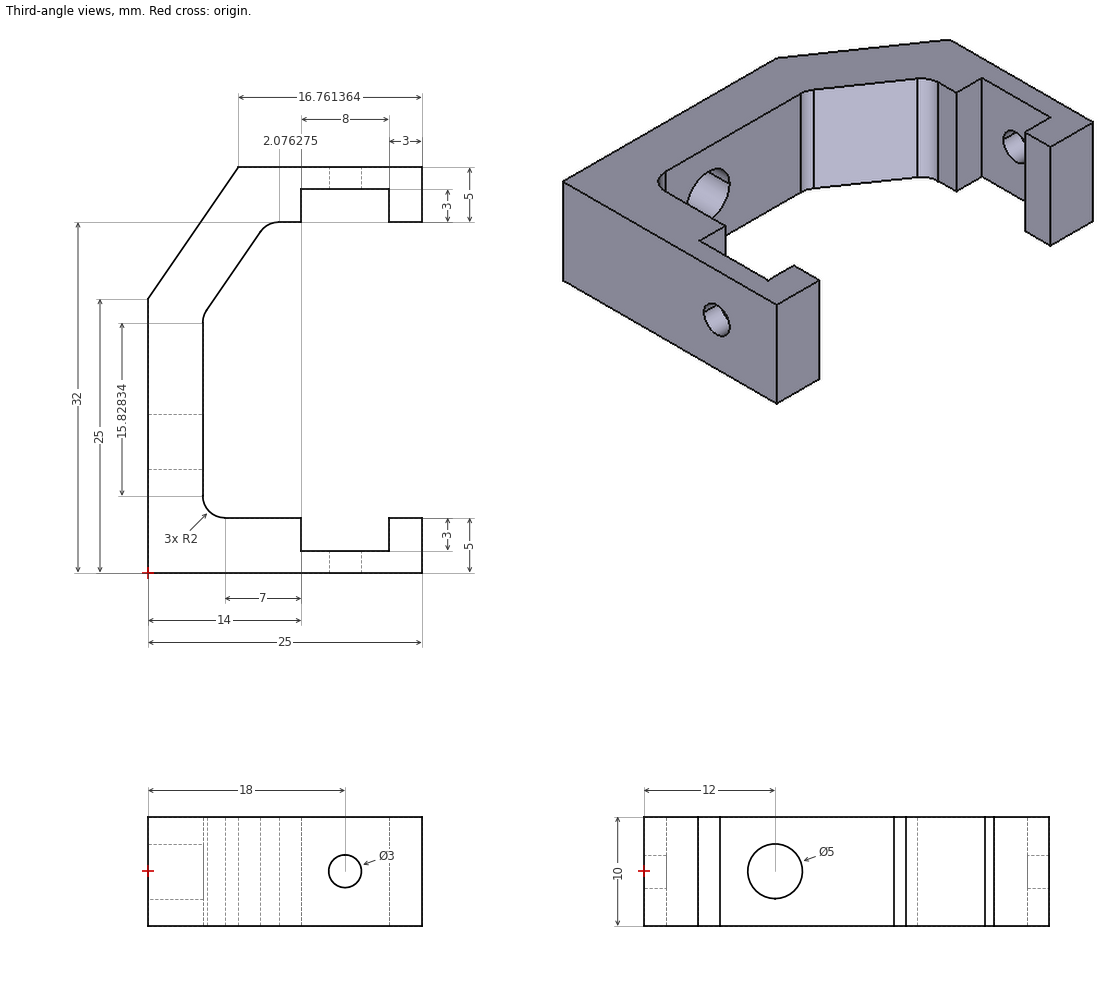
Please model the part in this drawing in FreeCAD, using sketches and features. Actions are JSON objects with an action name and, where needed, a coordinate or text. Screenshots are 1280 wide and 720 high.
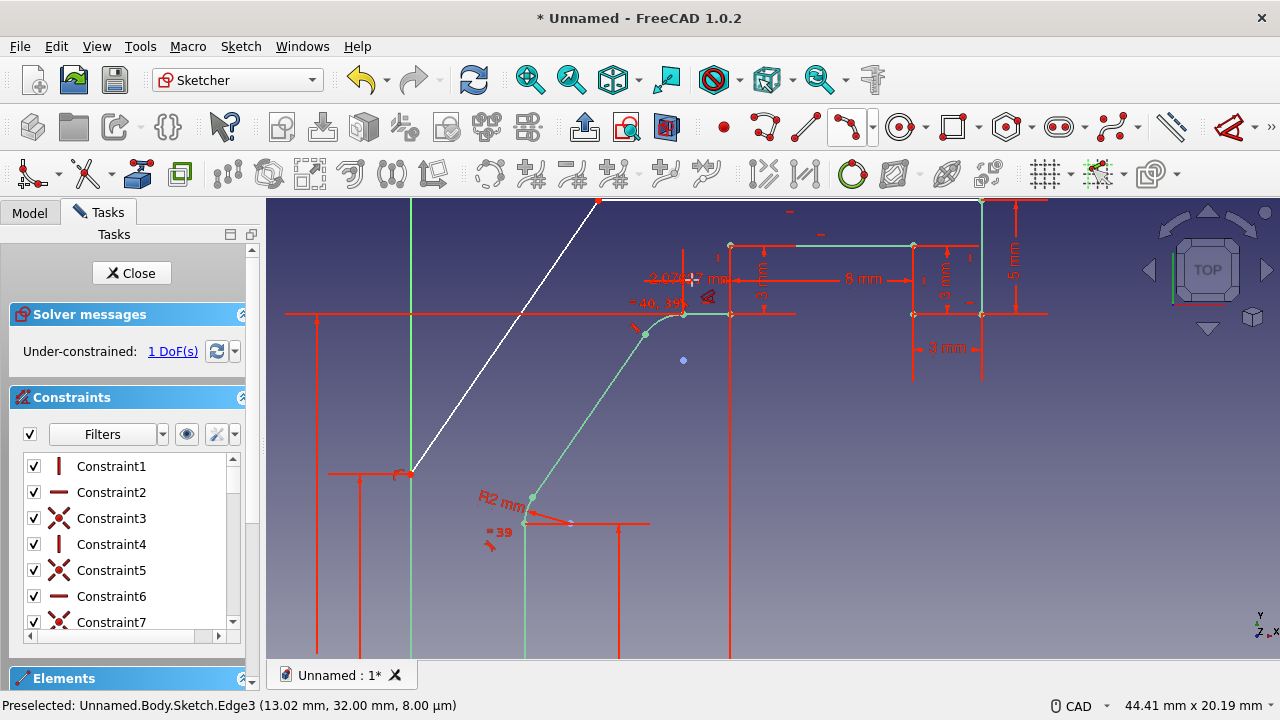
{"action": "scroll", "coordinate": [709, 316], "scroll_direction": "down", "scroll_amount": 5}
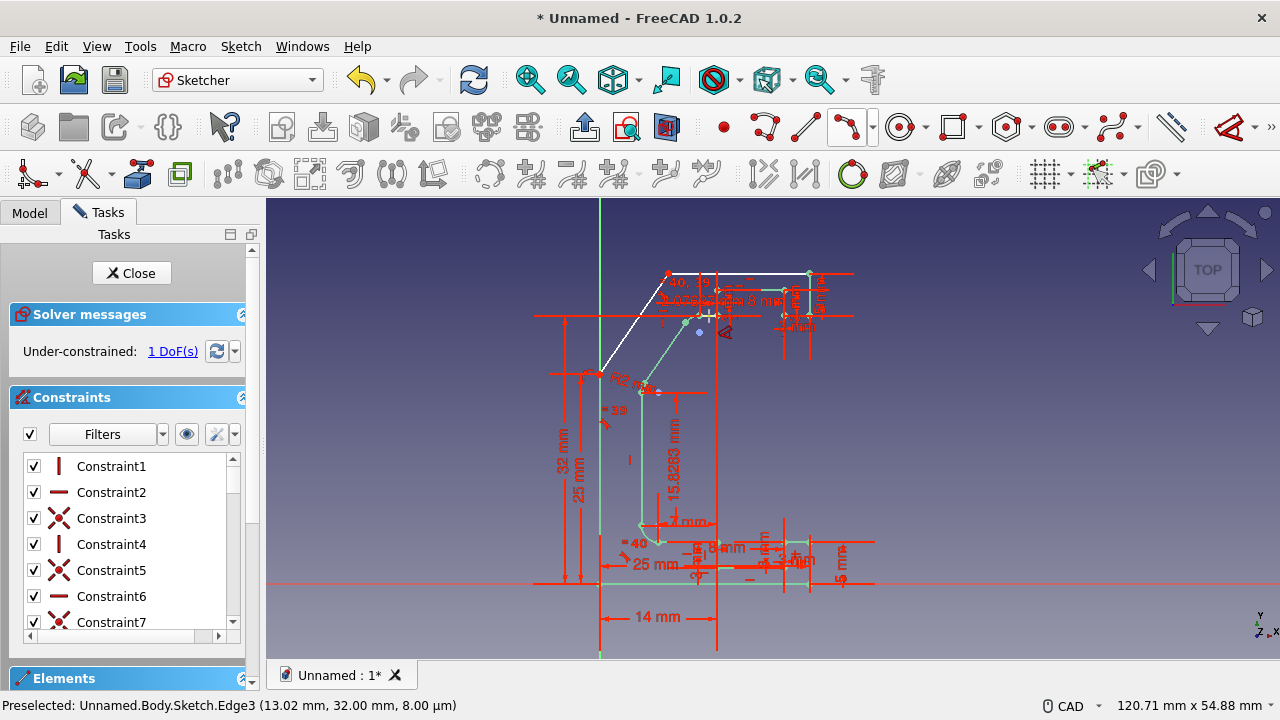
{"action": "left_click", "coordinate": [767, 274]}
{"action": "left_click", "coordinate": [739, 240]}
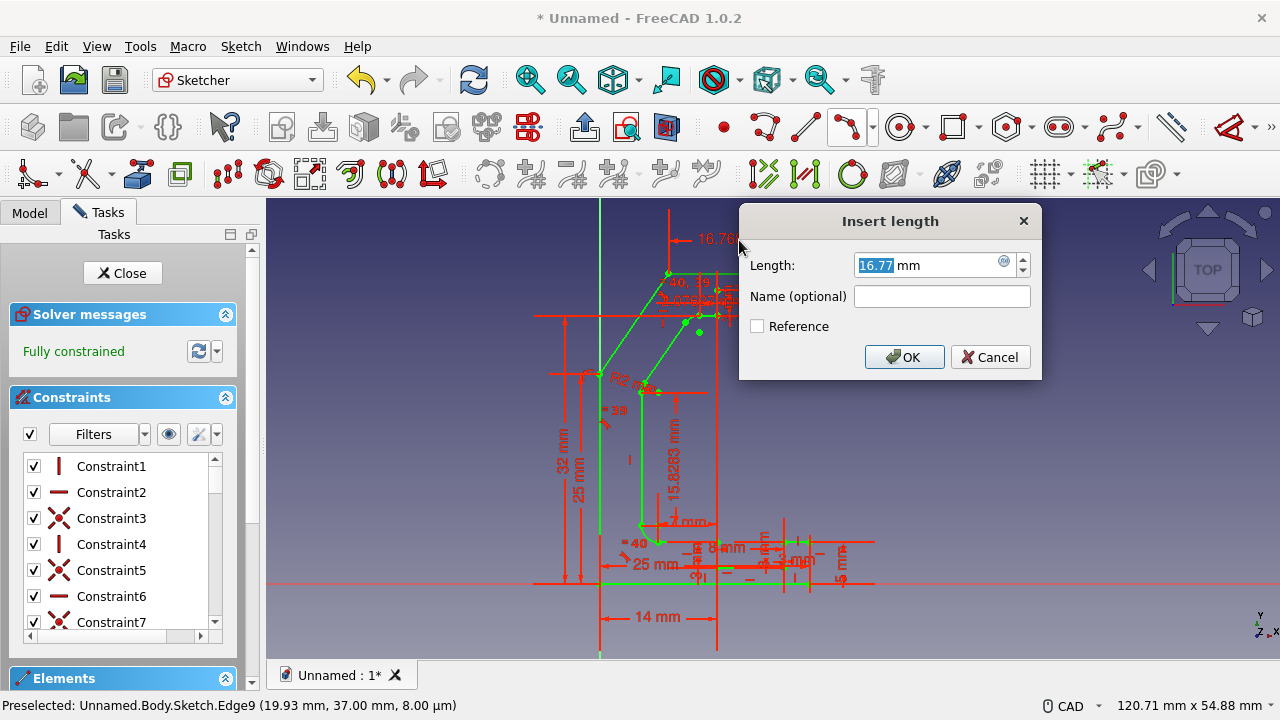
{"action": "type", "text": "16.761364"}
{"action": "key", "text": "Return"}
{"action": "key", "text": "Escape"}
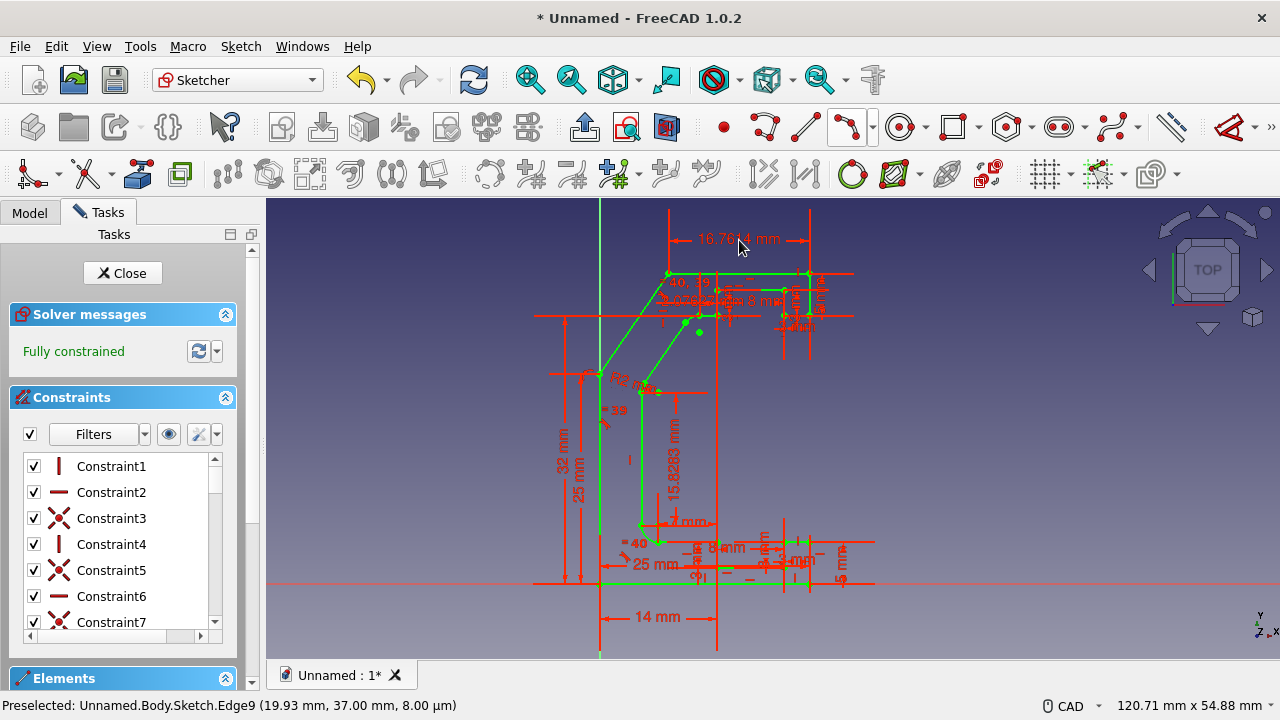
{"action": "left_click", "coordinate": [123, 273]}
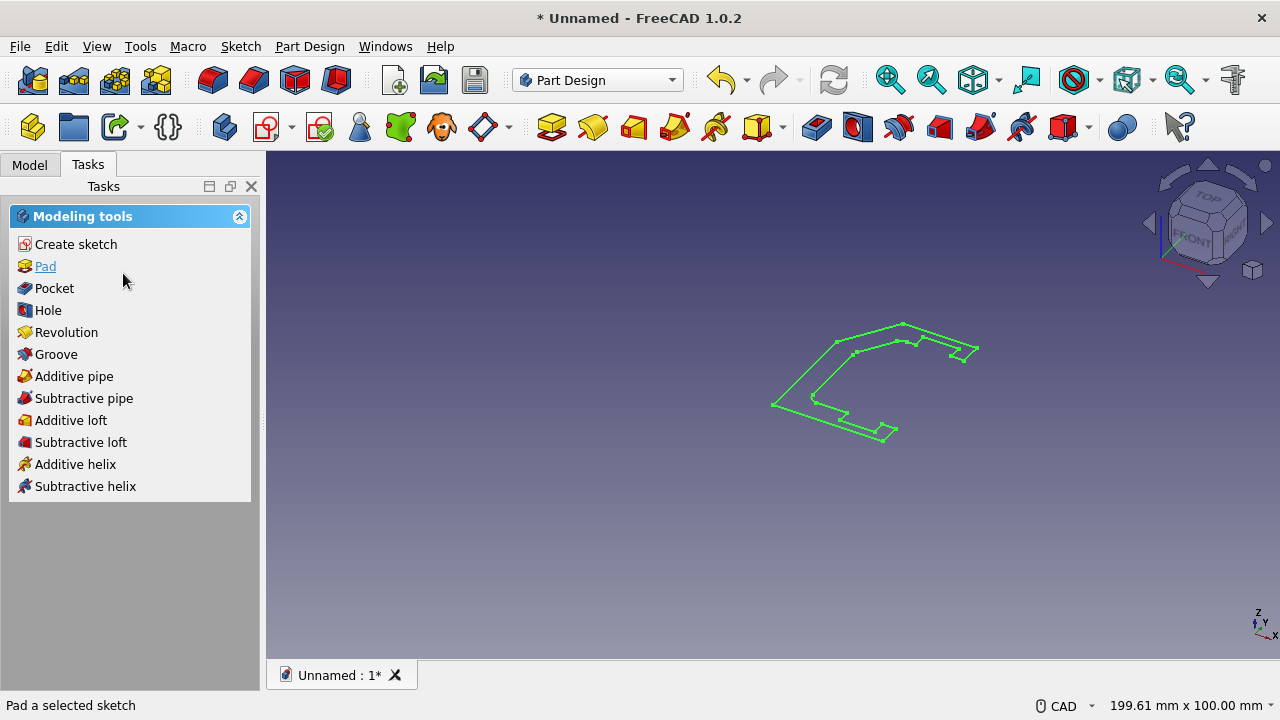
{"action": "left_click", "coordinate": [552, 128]}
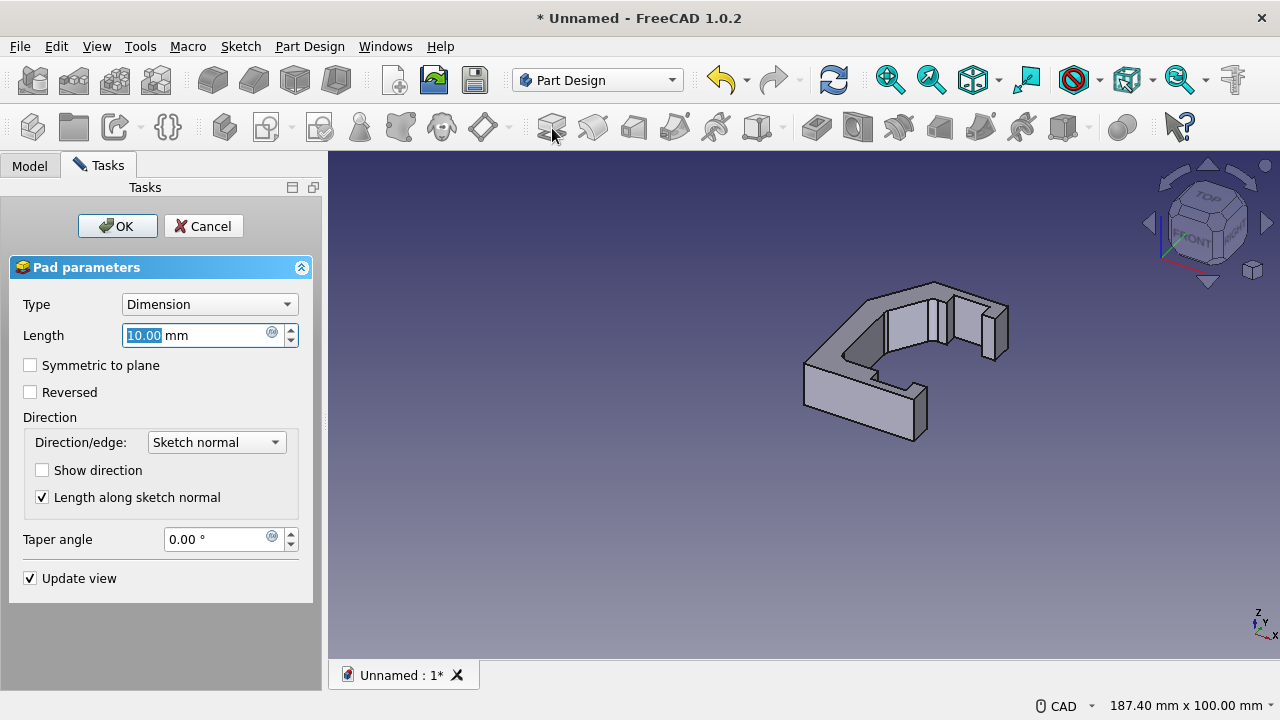
{"action": "type", "text": "10"}
{"action": "key", "text": "Tab"}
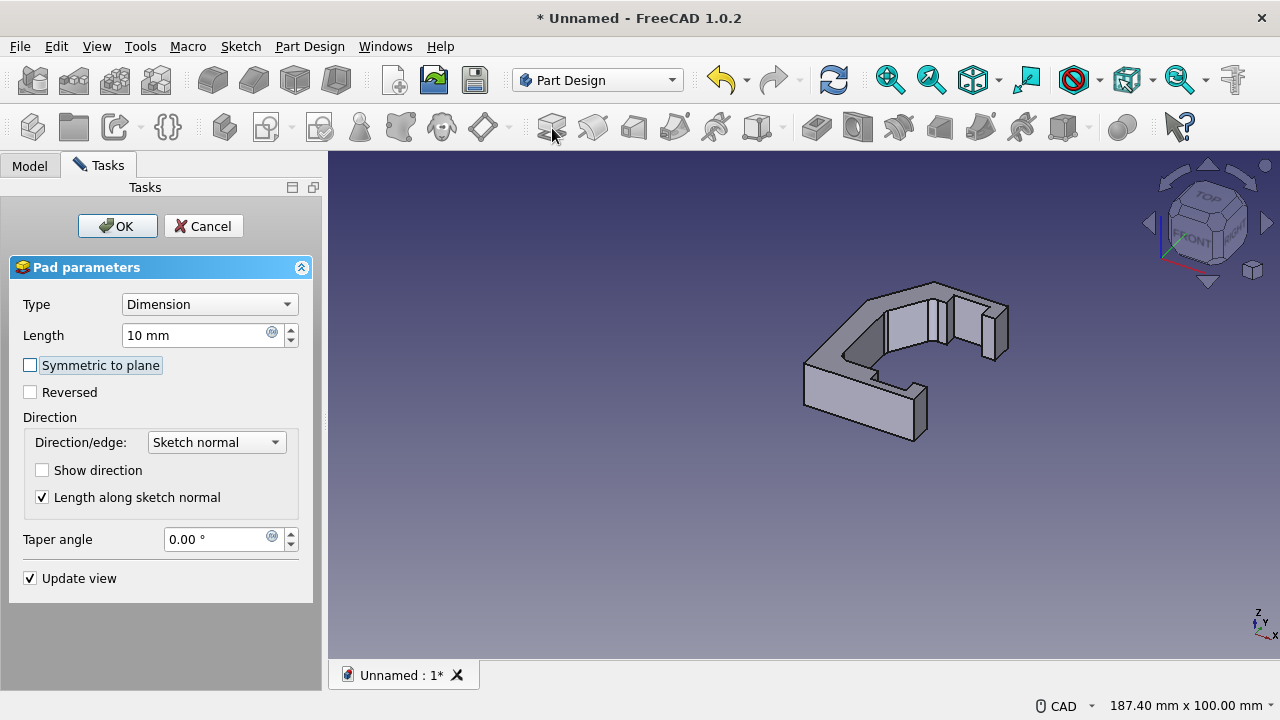
{"action": "left_click", "coordinate": [31, 365]}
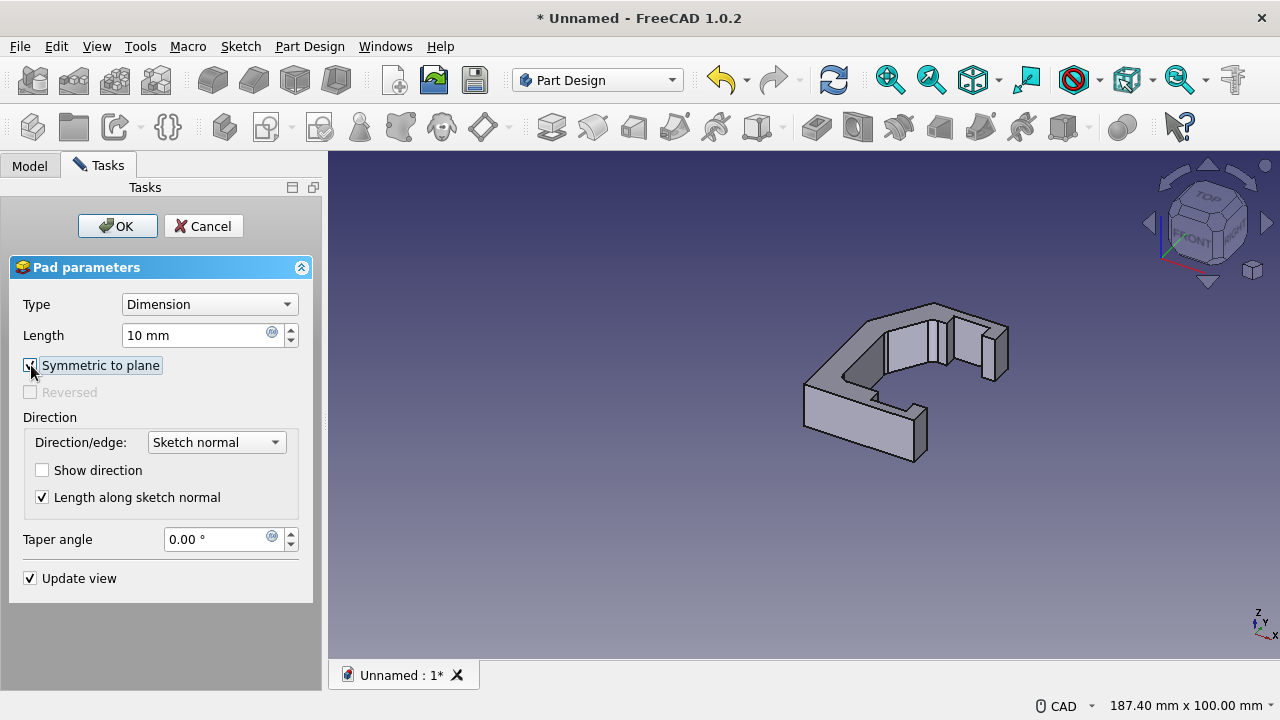
{"action": "left_click", "coordinate": [118, 226]}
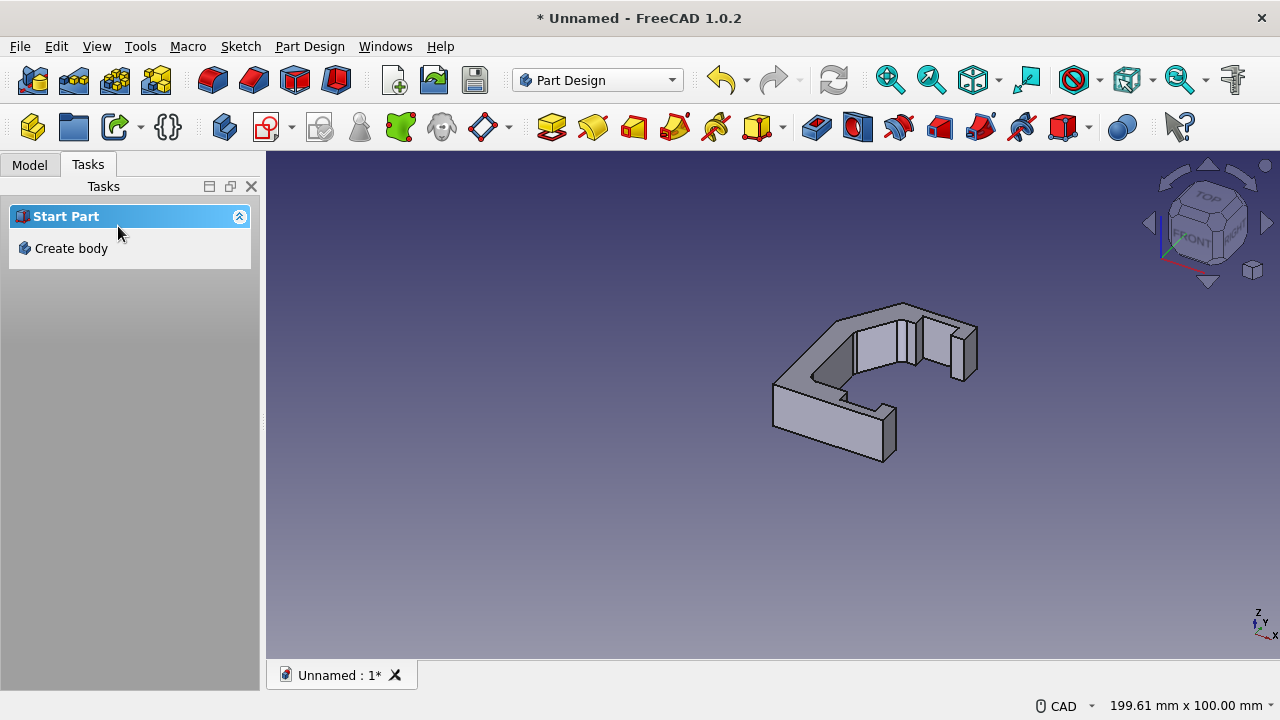
{"action": "left_click", "coordinate": [891, 80]}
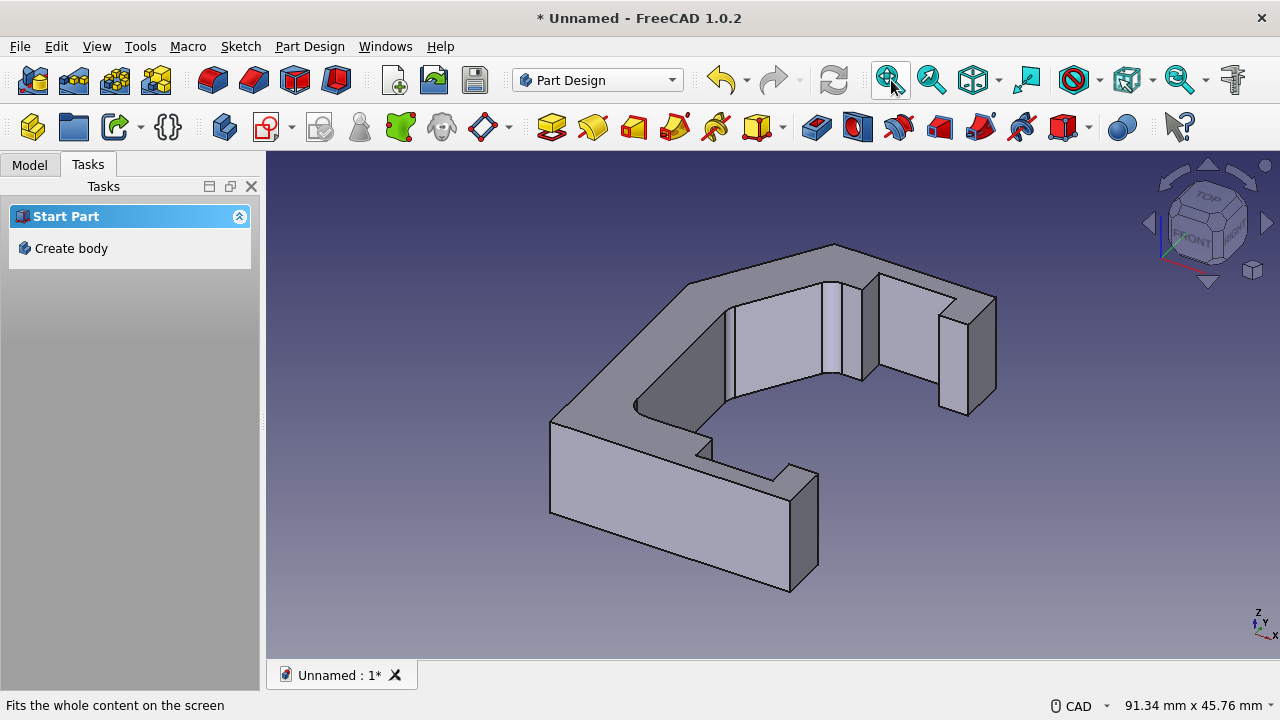
{"action": "left_click", "coordinate": [694, 387]}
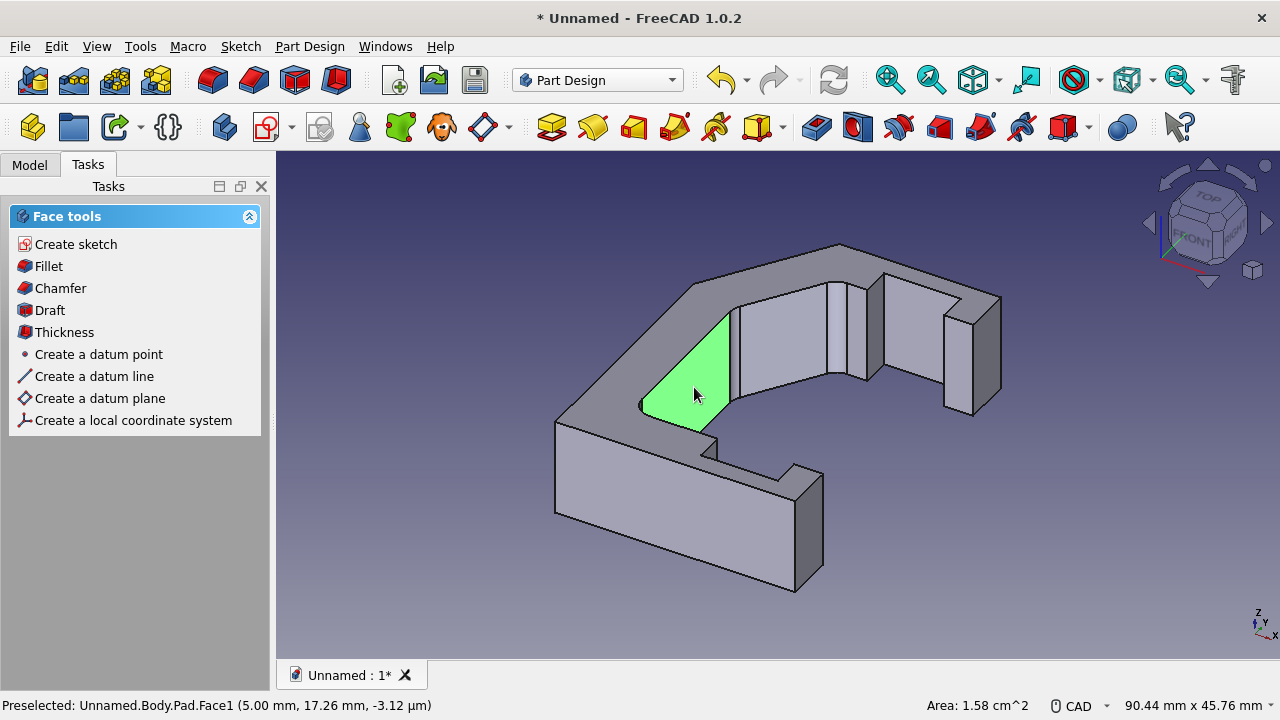
{"action": "left_click", "coordinate": [266, 128]}